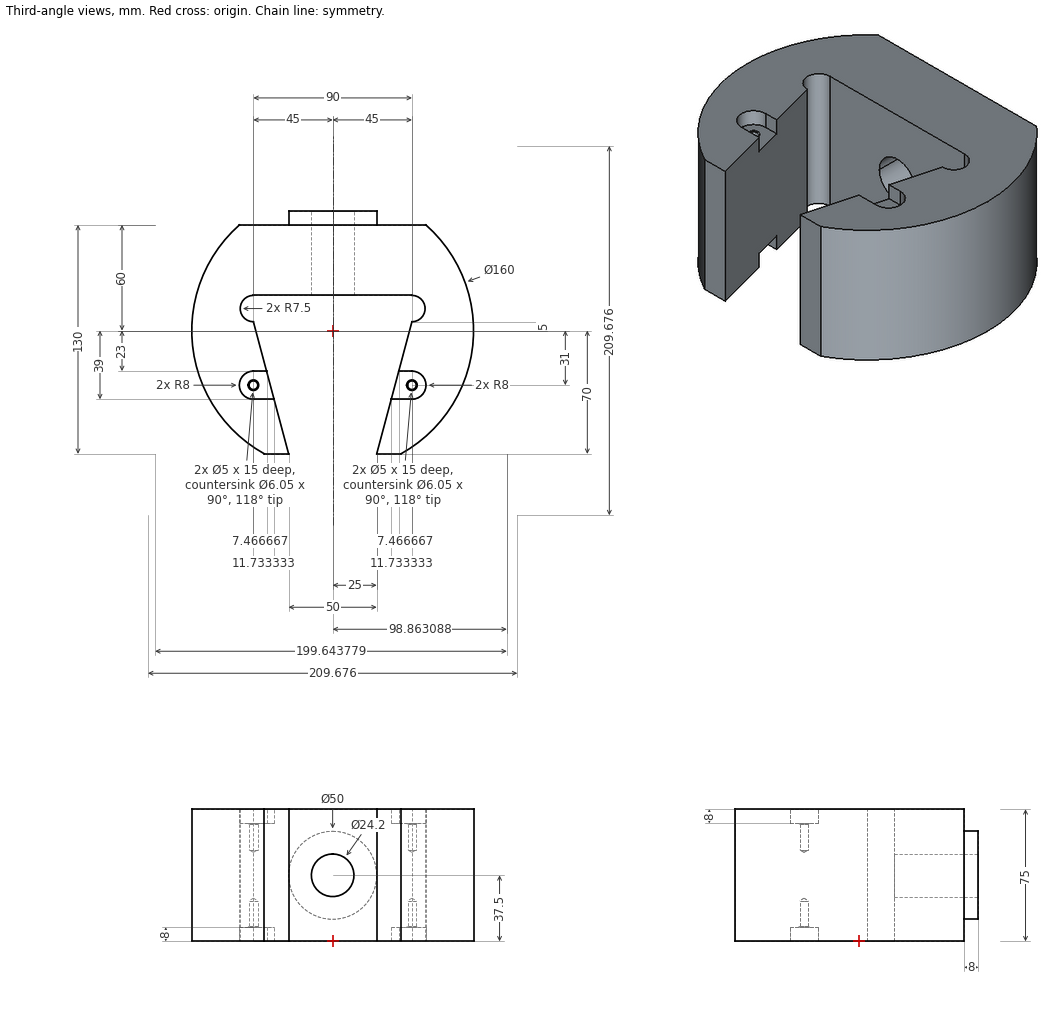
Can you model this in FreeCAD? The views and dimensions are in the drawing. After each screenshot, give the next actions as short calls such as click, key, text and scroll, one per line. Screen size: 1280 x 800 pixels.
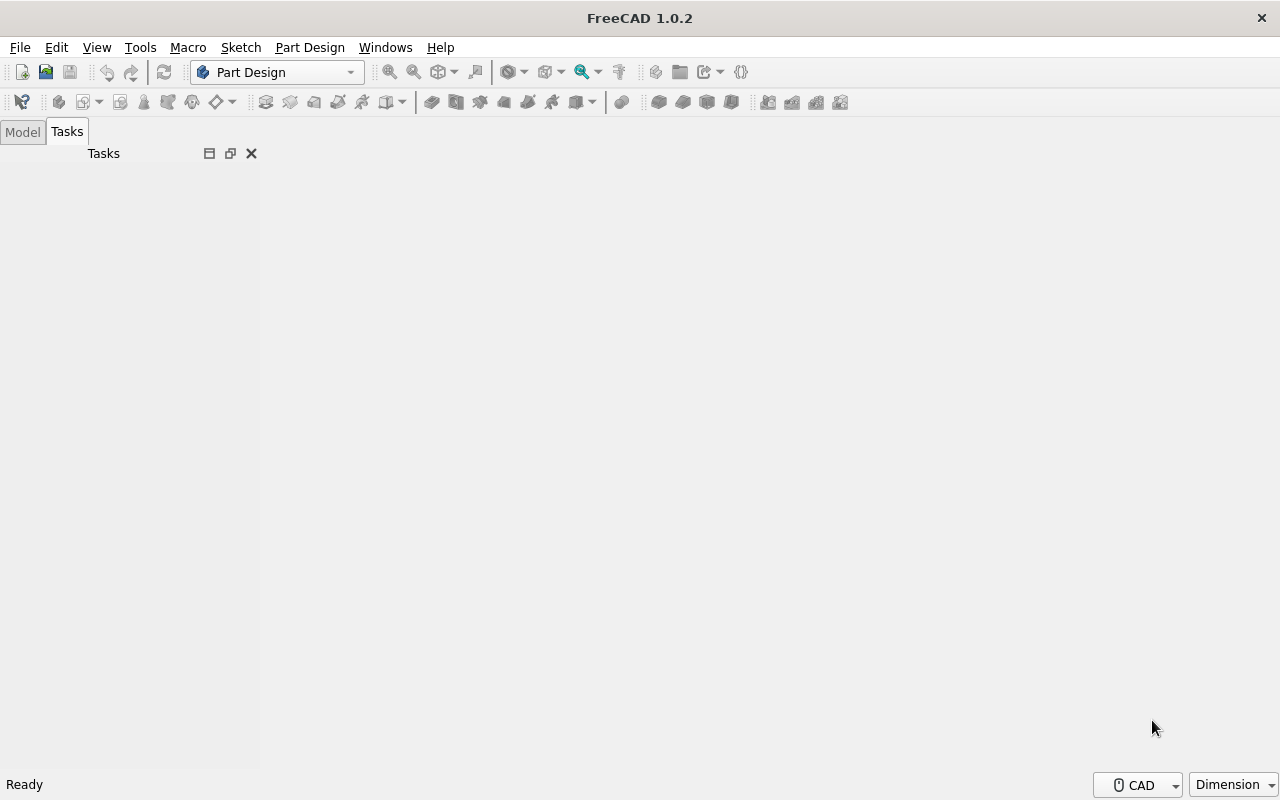
key(ctrl+n)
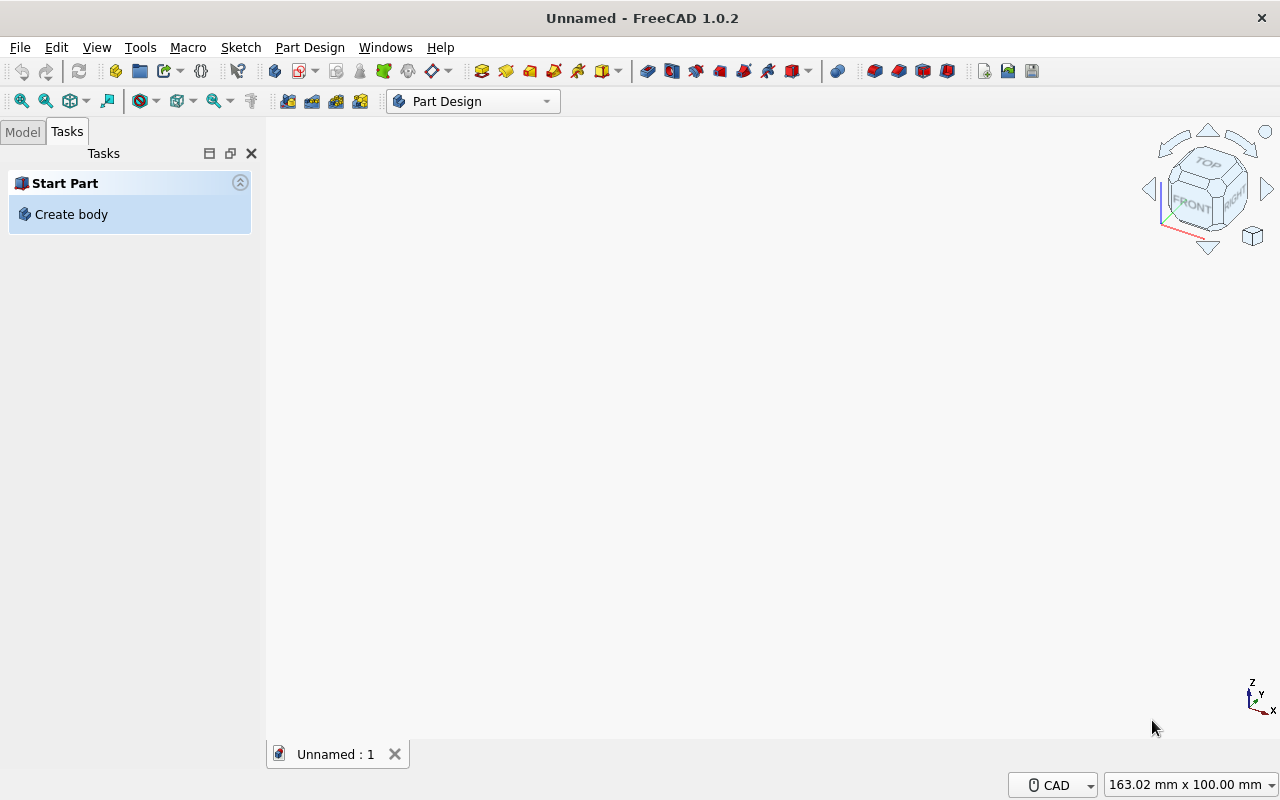
click(300, 72)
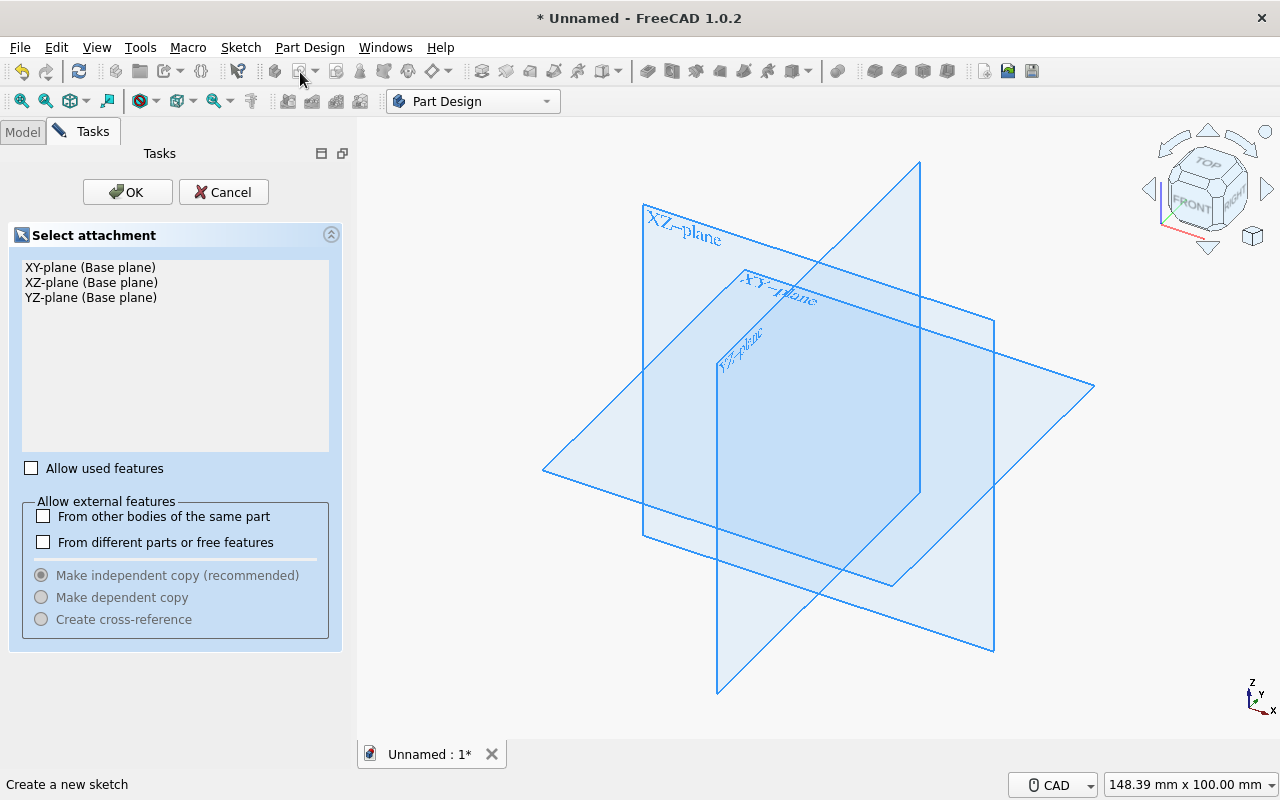
click(82, 268)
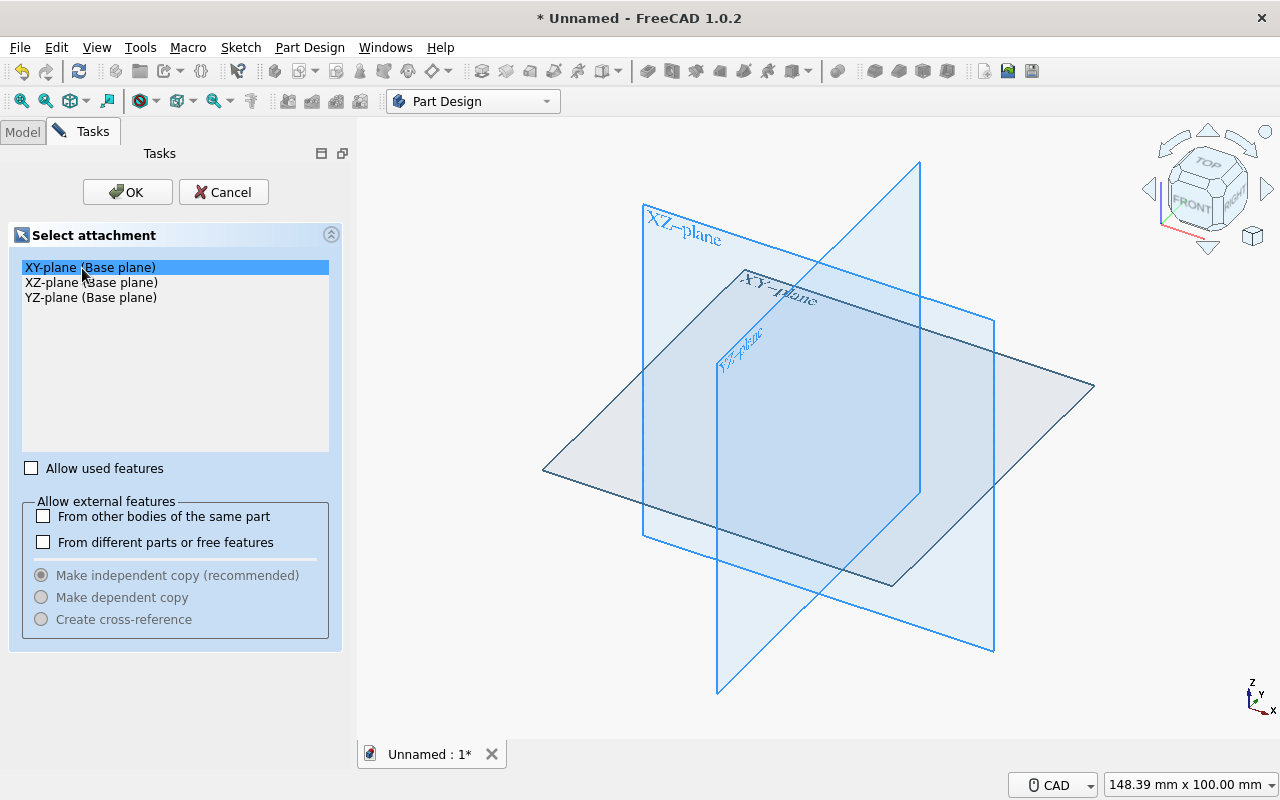
click(128, 192)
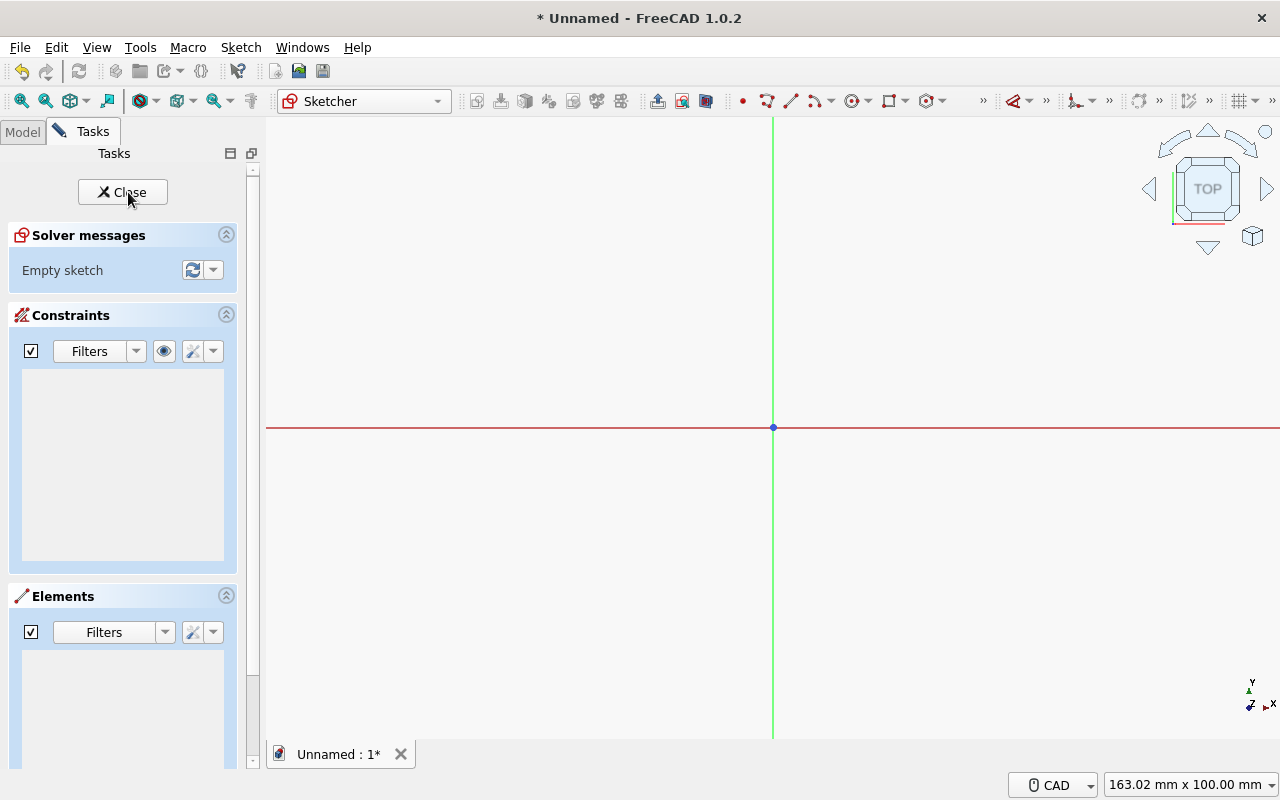
scroll(665, 428, down, 5)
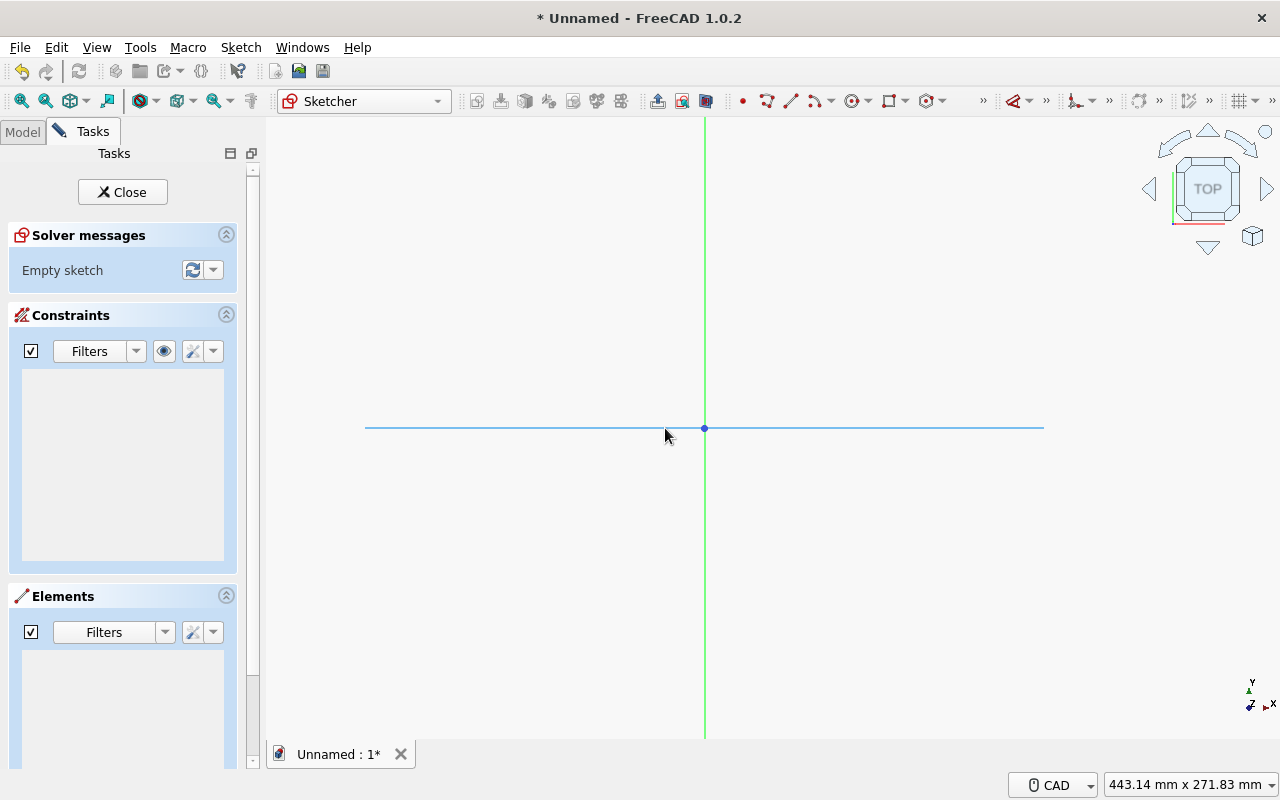
key(g)
key(c)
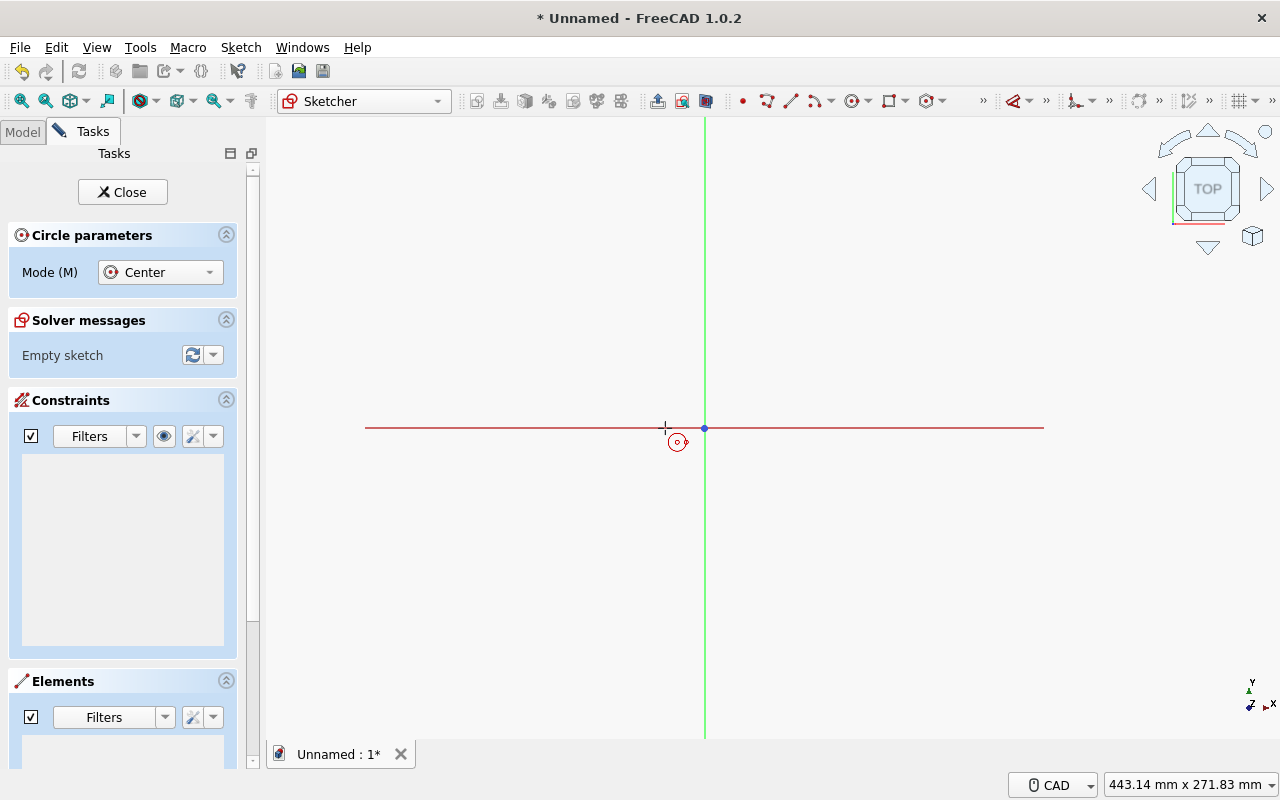
click(705, 428)
move(834, 299)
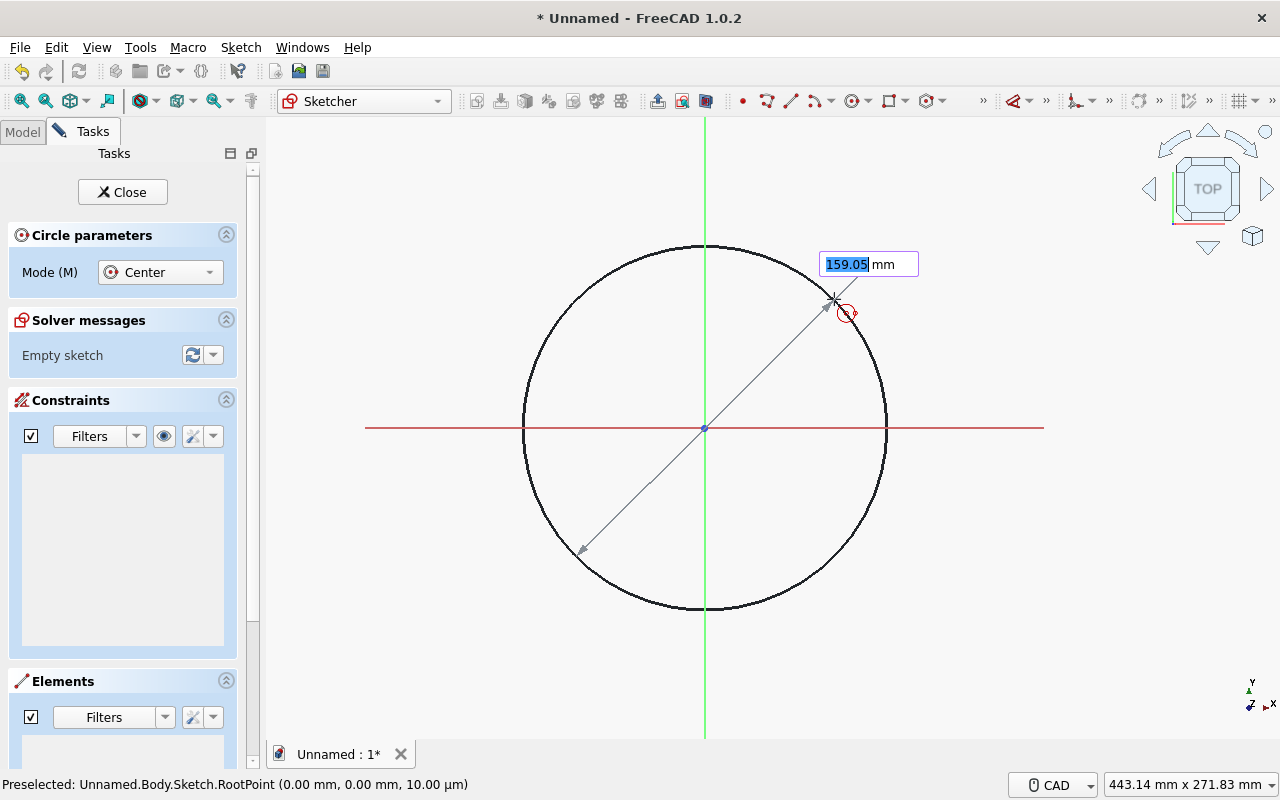
text(160)
key(Return)
key(Escape)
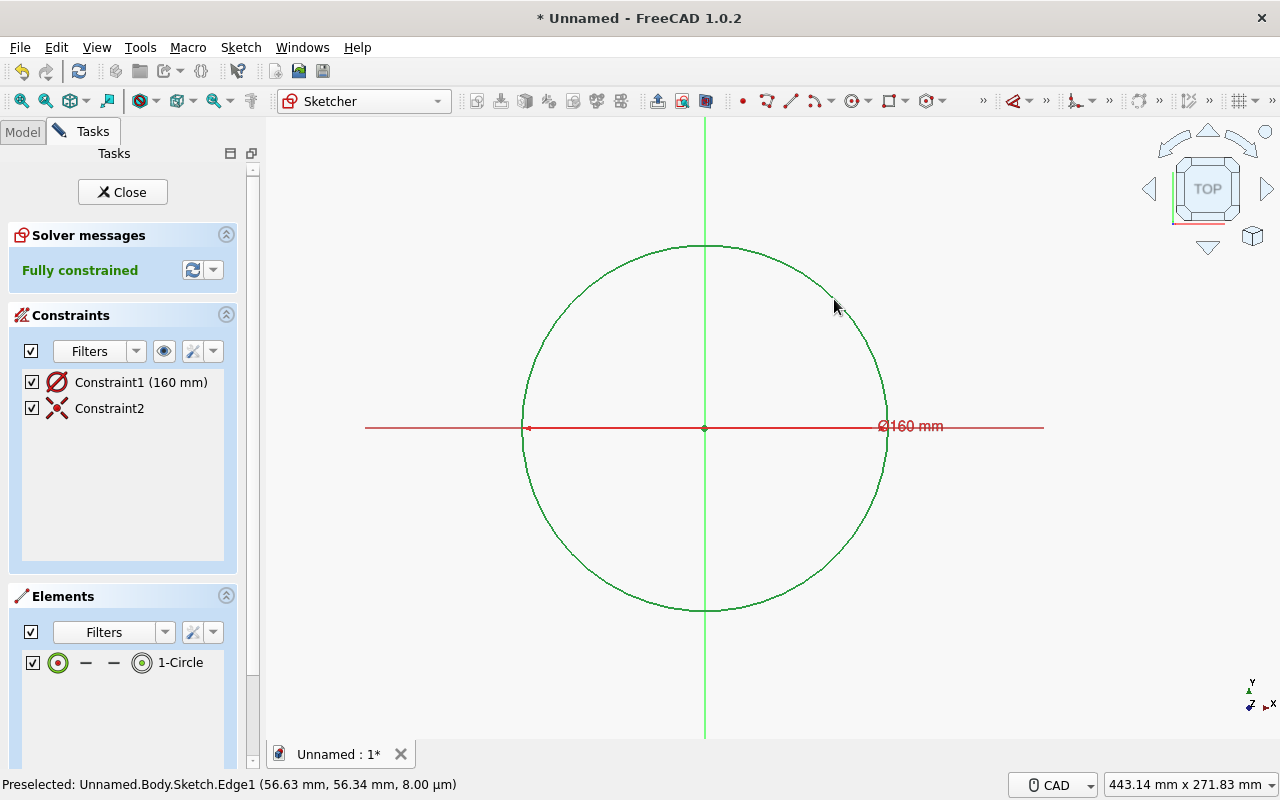
click(123, 192)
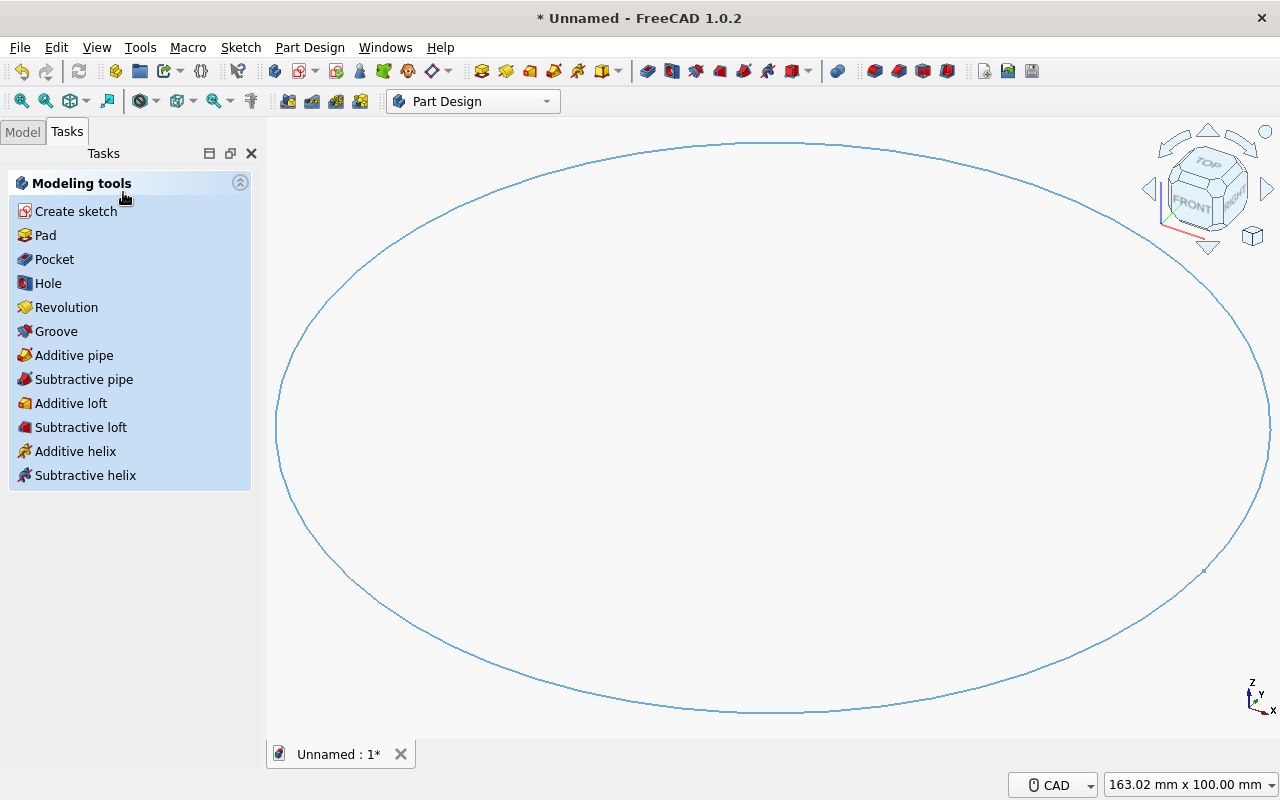
click(482, 72)